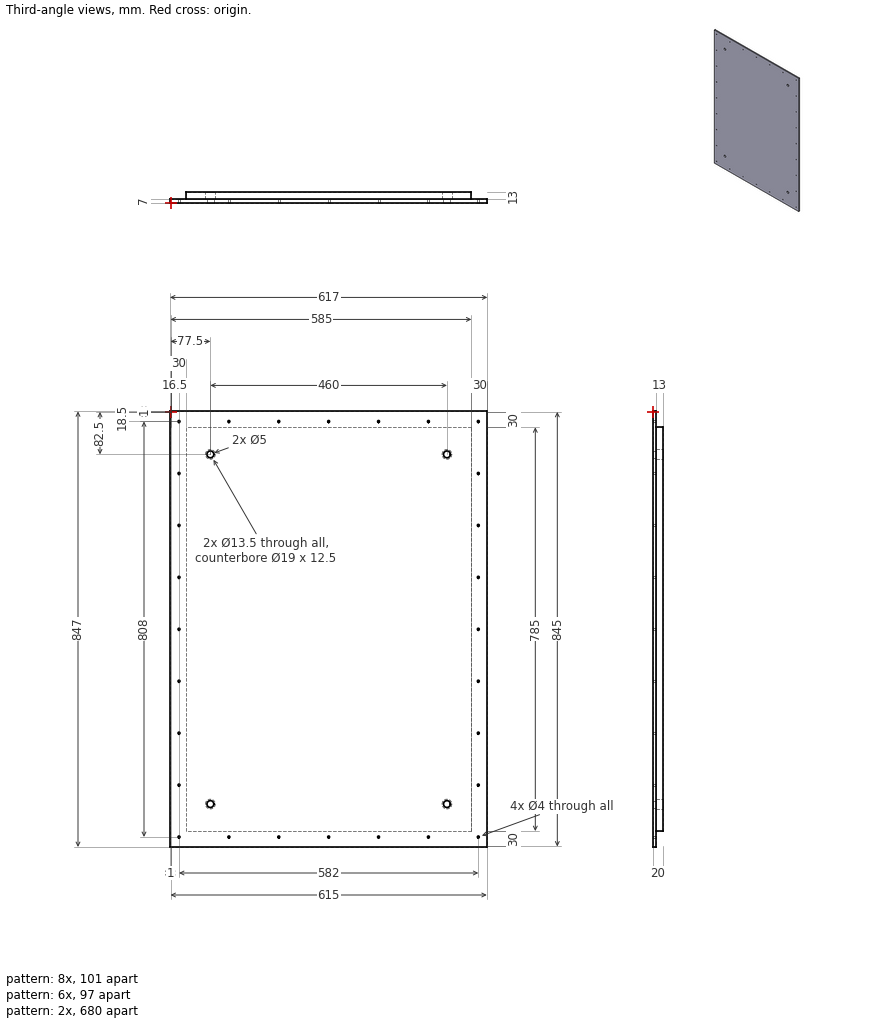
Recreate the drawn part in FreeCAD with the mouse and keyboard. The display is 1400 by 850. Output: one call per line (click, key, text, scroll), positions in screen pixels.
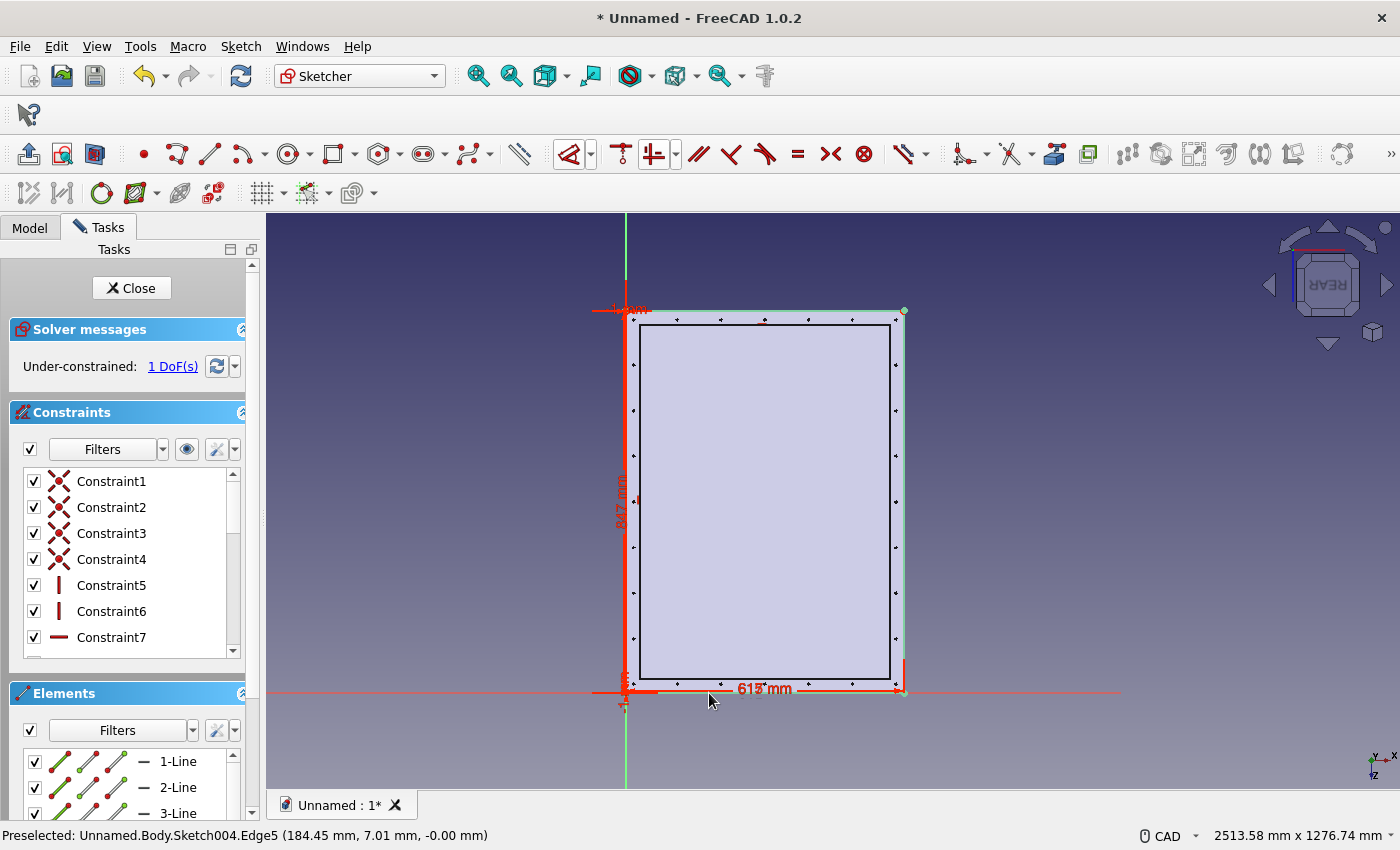
scroll(904, 578, up, 15)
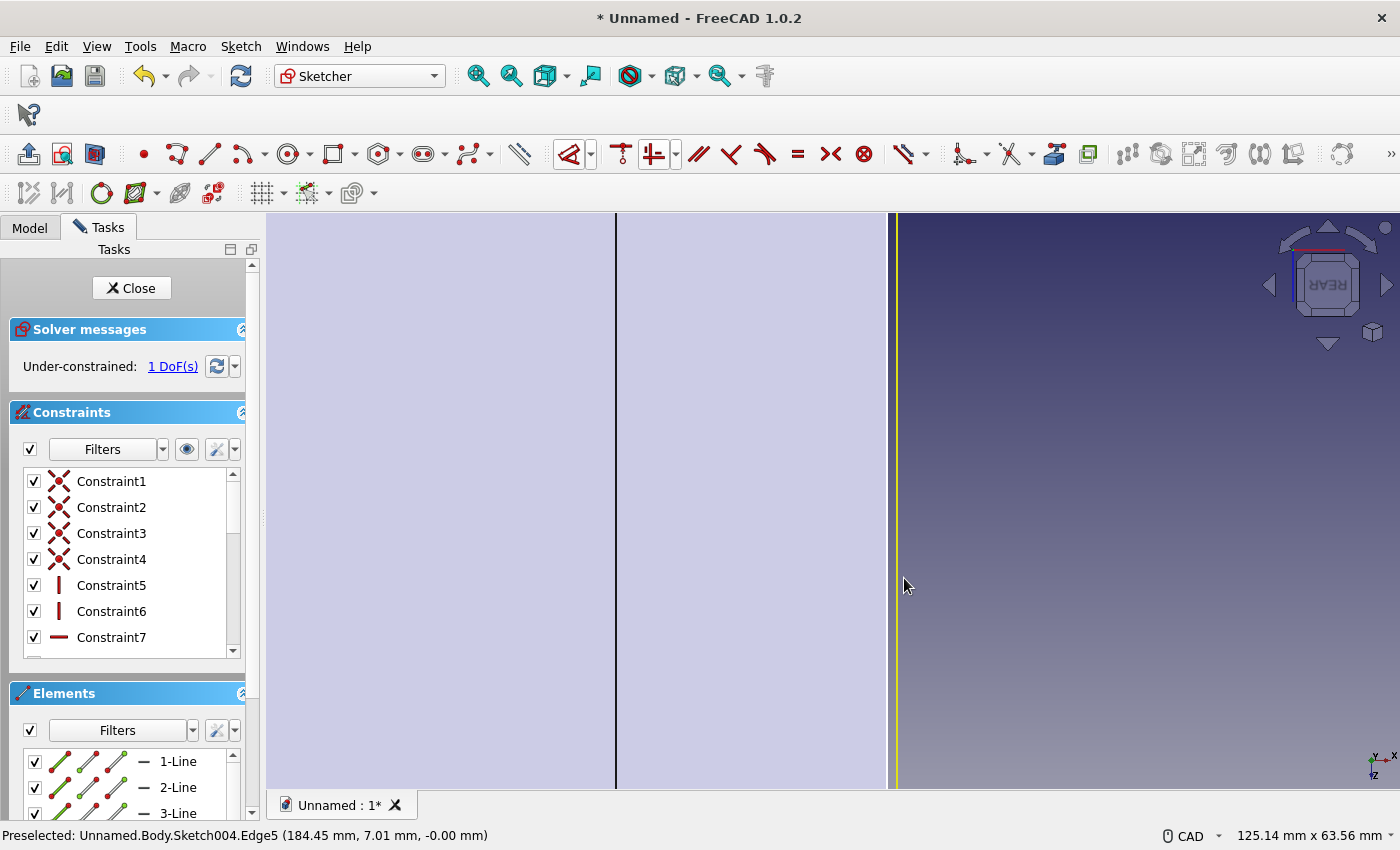
click(887, 570)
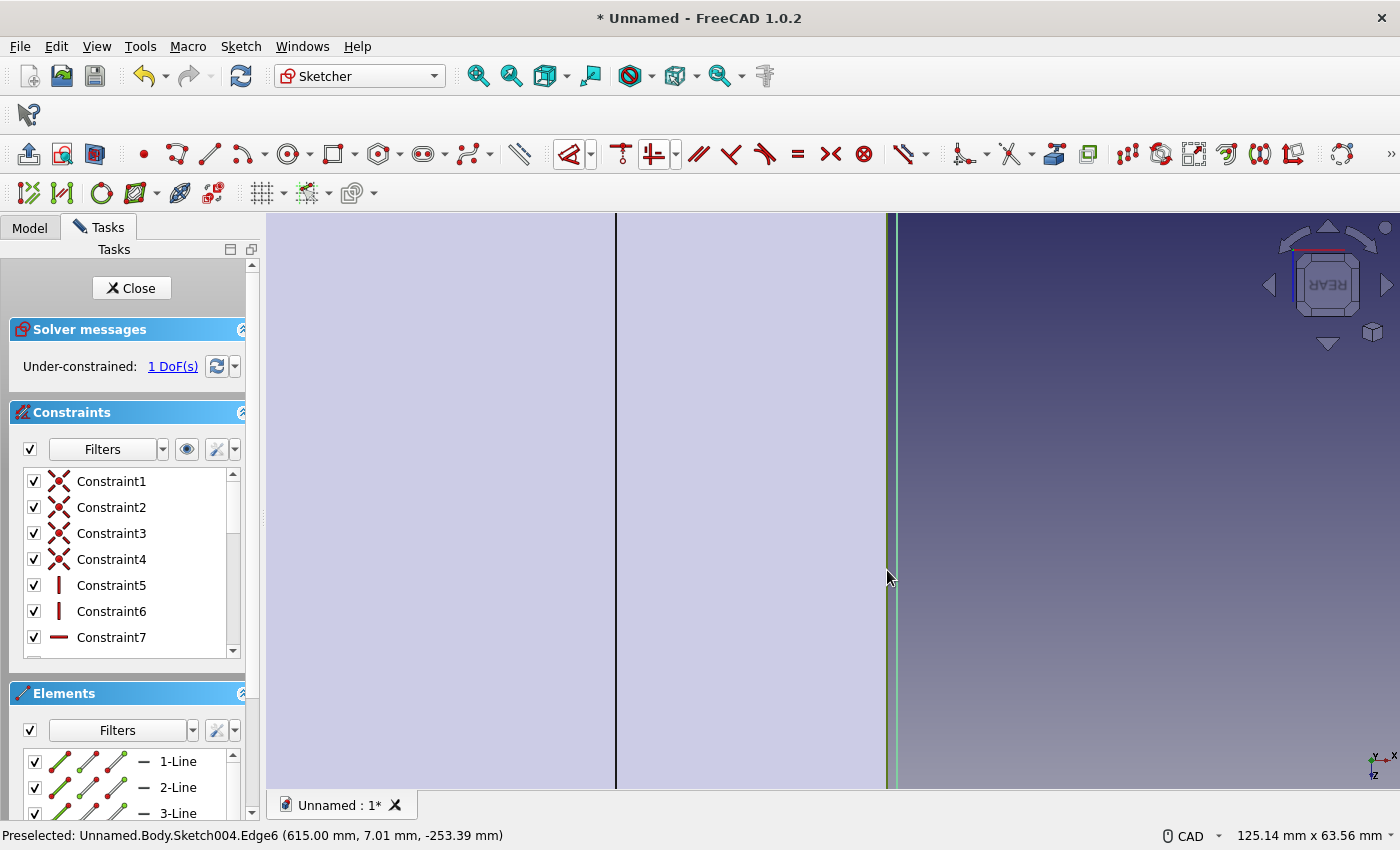
click(590, 154)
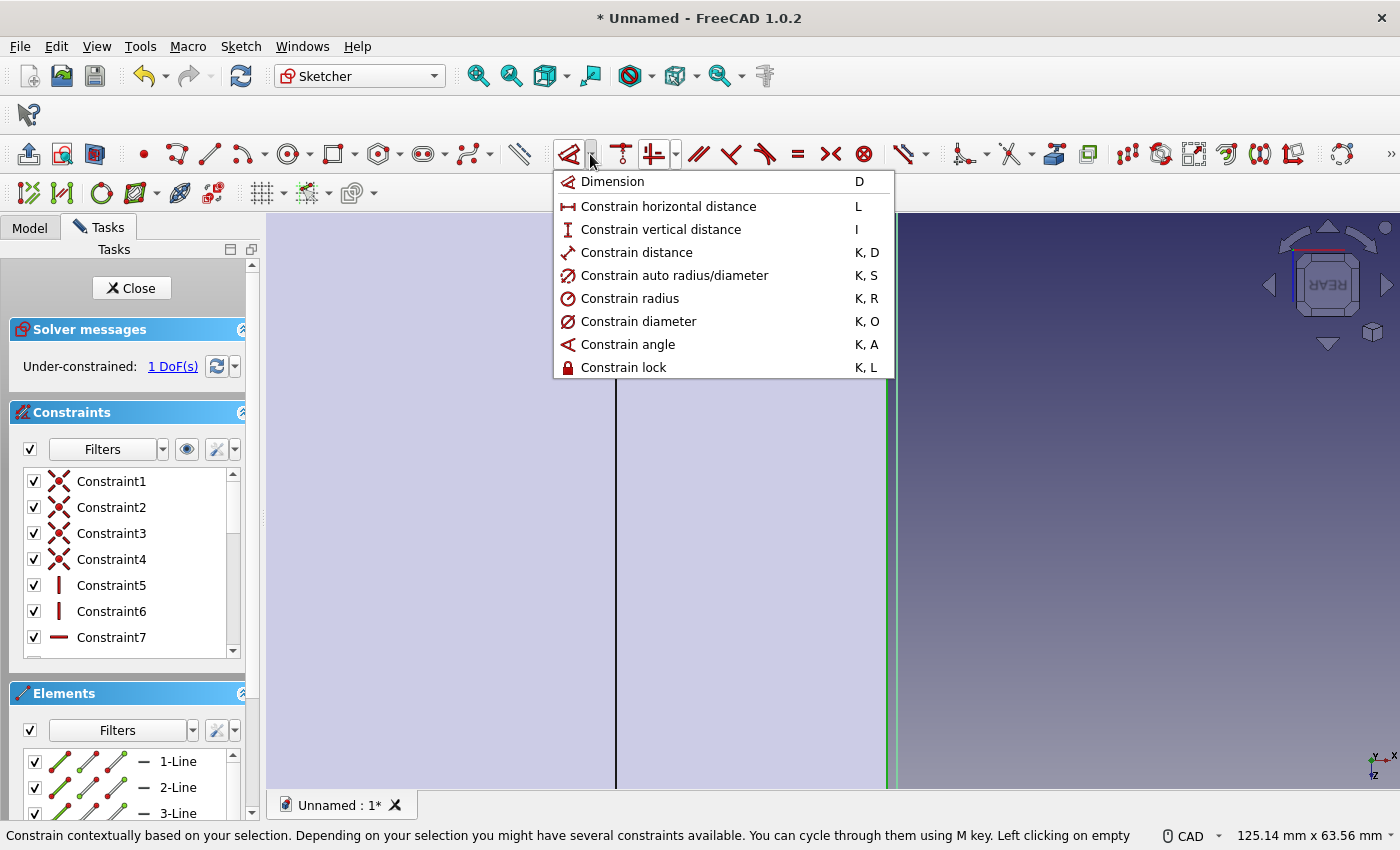
click(724, 230)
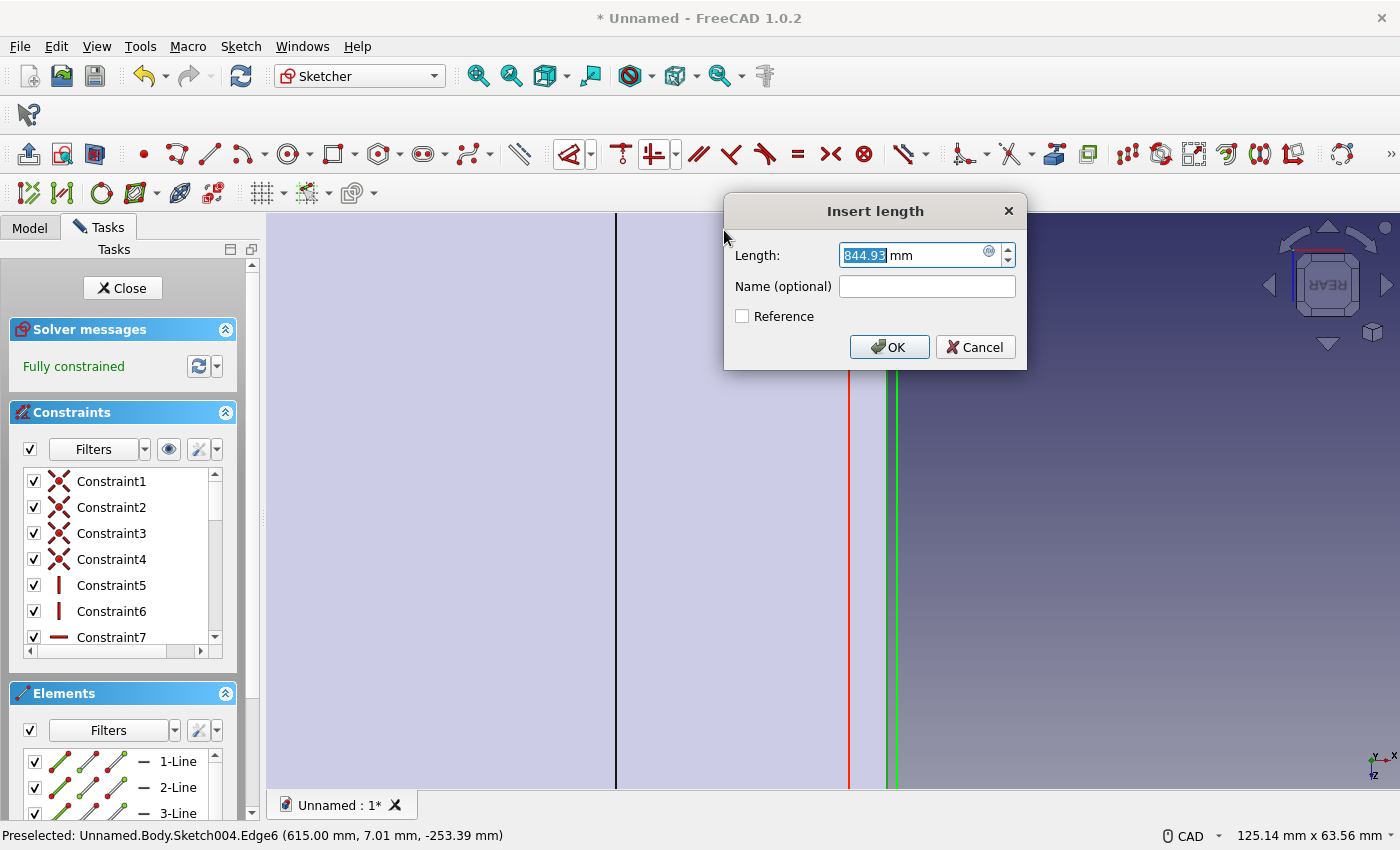
text(845)
key(Return)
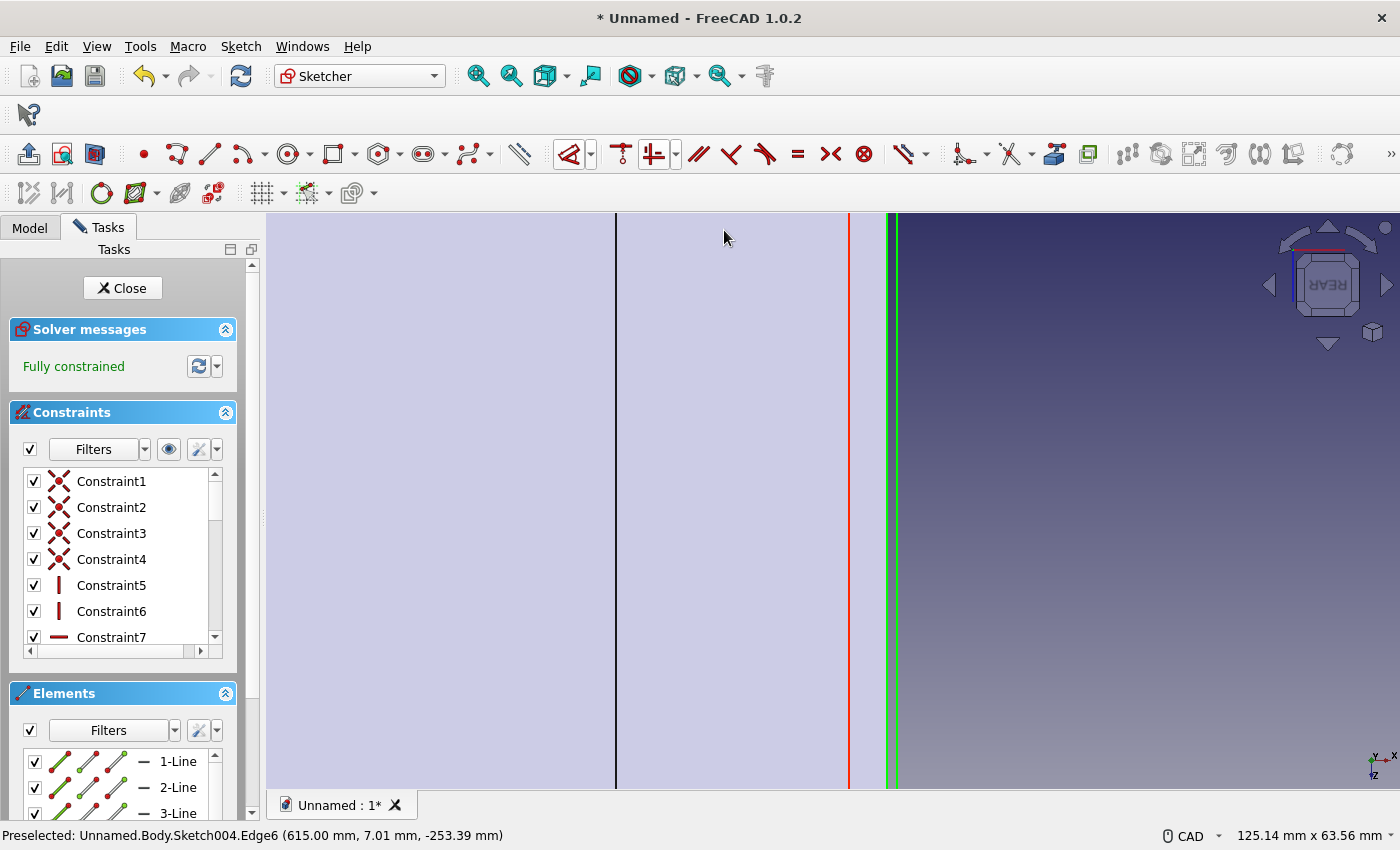
click(123, 288)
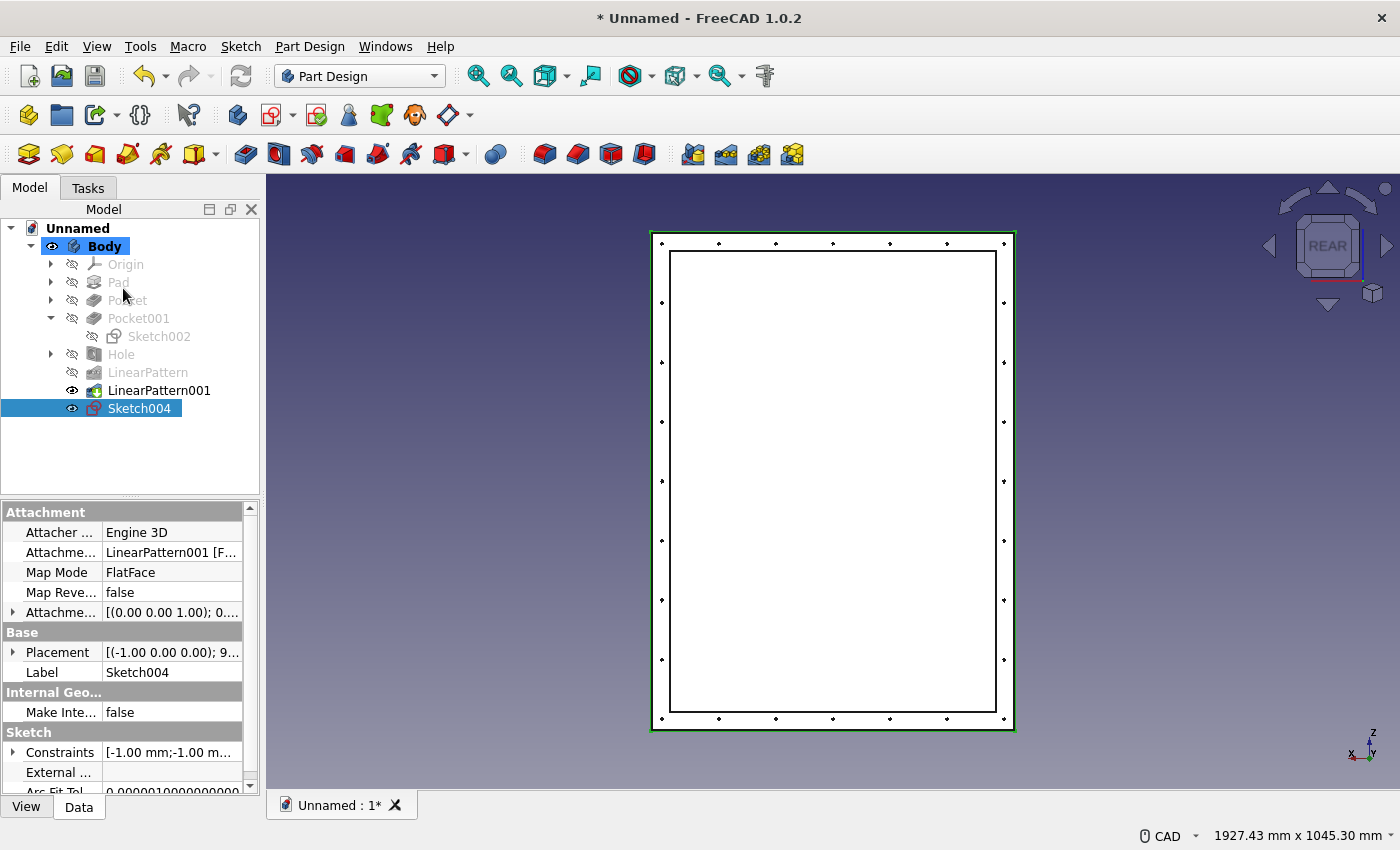
click(29, 154)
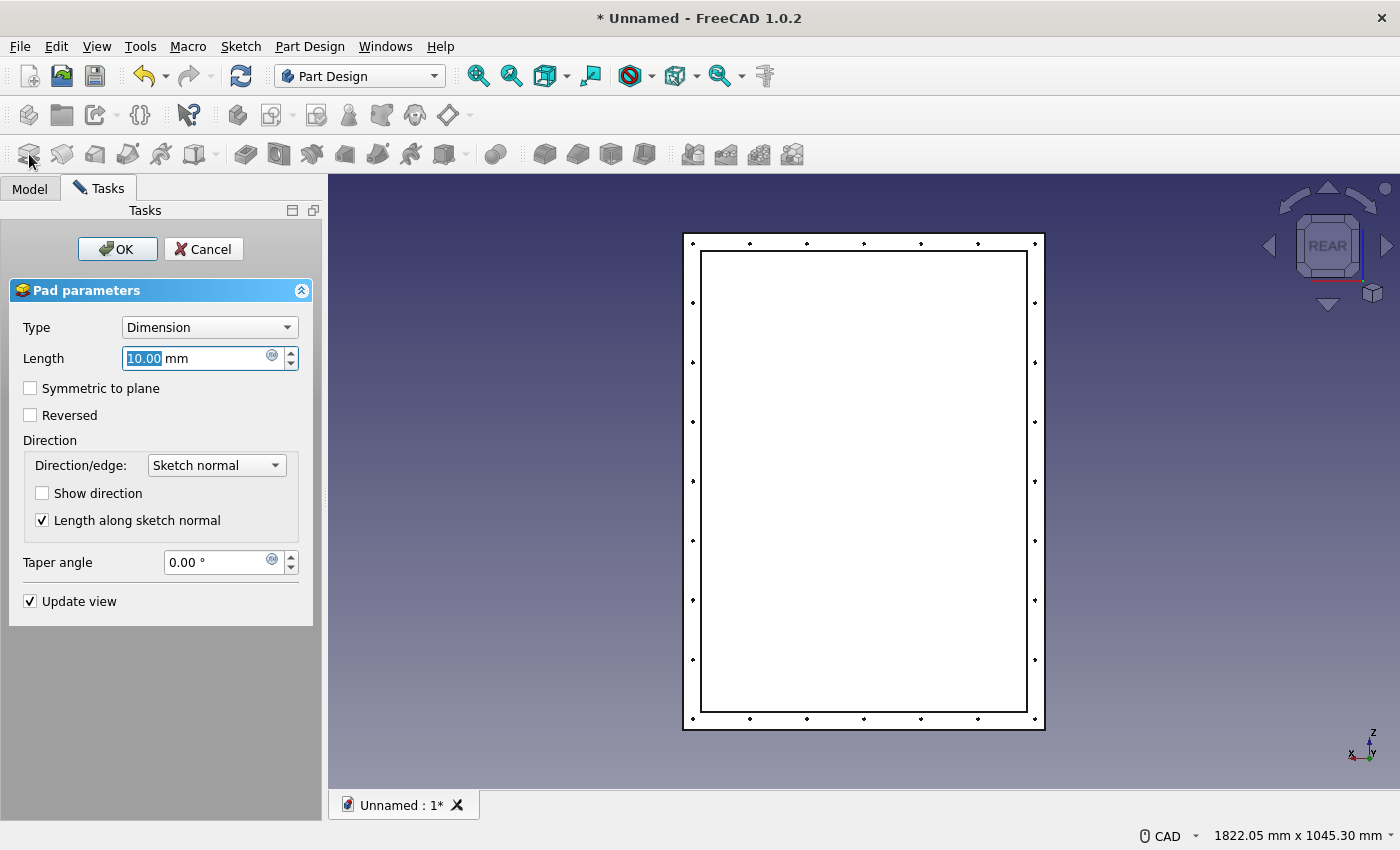
text(7)
key(Tab)